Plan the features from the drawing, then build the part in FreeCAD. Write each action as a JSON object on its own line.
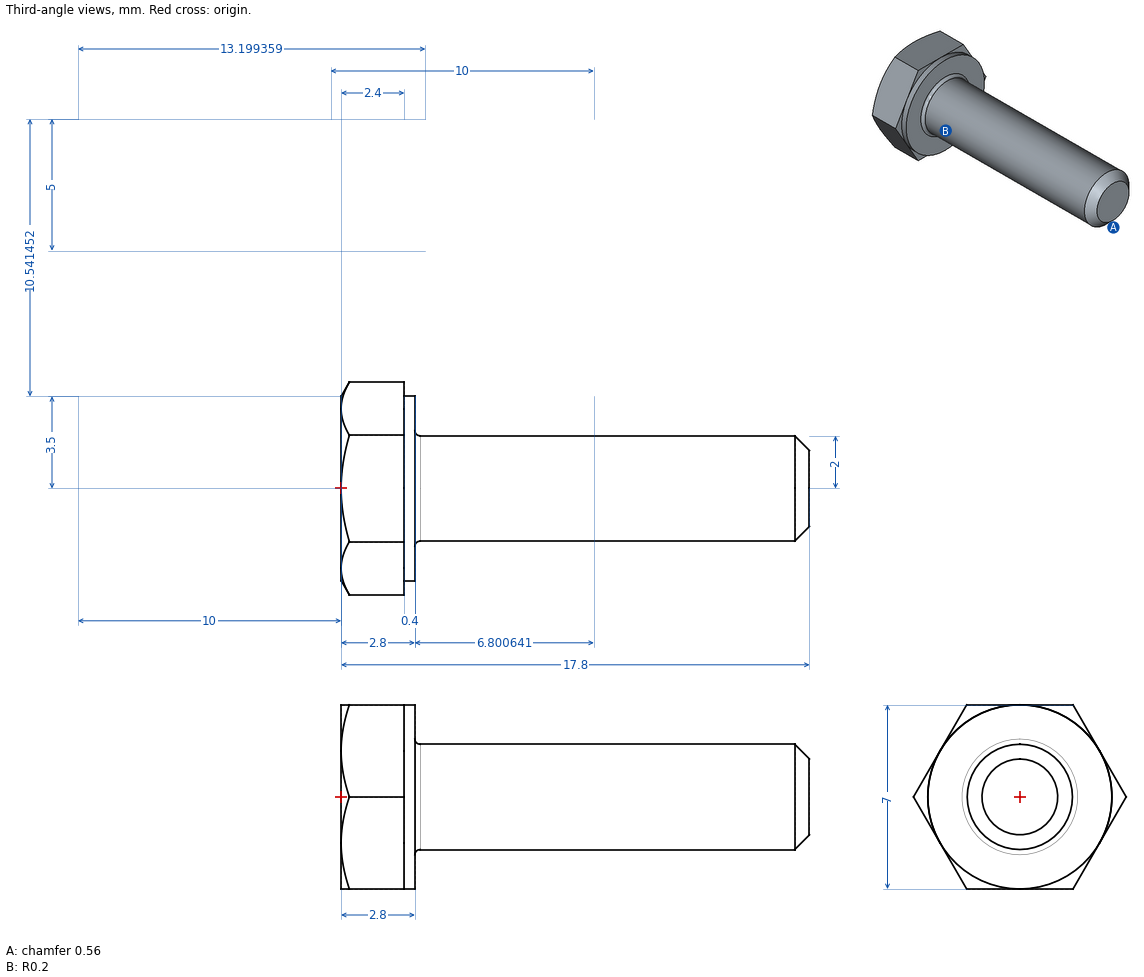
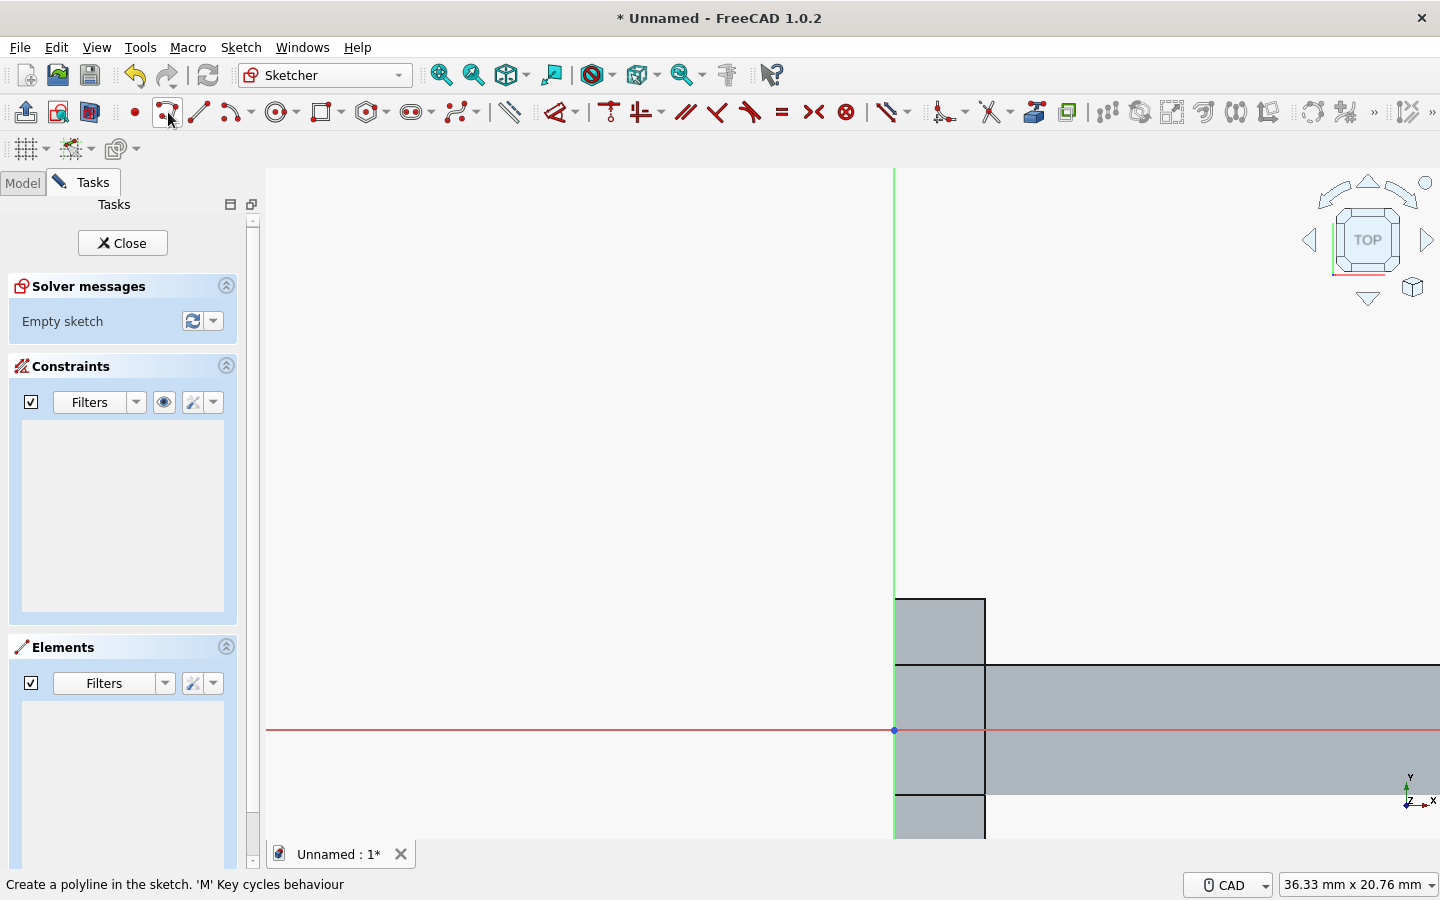
{"action": "left_click", "coordinate": [894, 617]}
{"action": "left_click", "coordinate": [998, 438]}
{"action": "left_click", "coordinate": [998, 276]}
{"action": "left_click", "coordinate": [571, 276]}
{"action": "left_click", "coordinate": [571, 617]}
{"action": "left_click", "coordinate": [894, 618]}
{"action": "key", "text": "Escape"}
{"action": "key", "text": "Escape"}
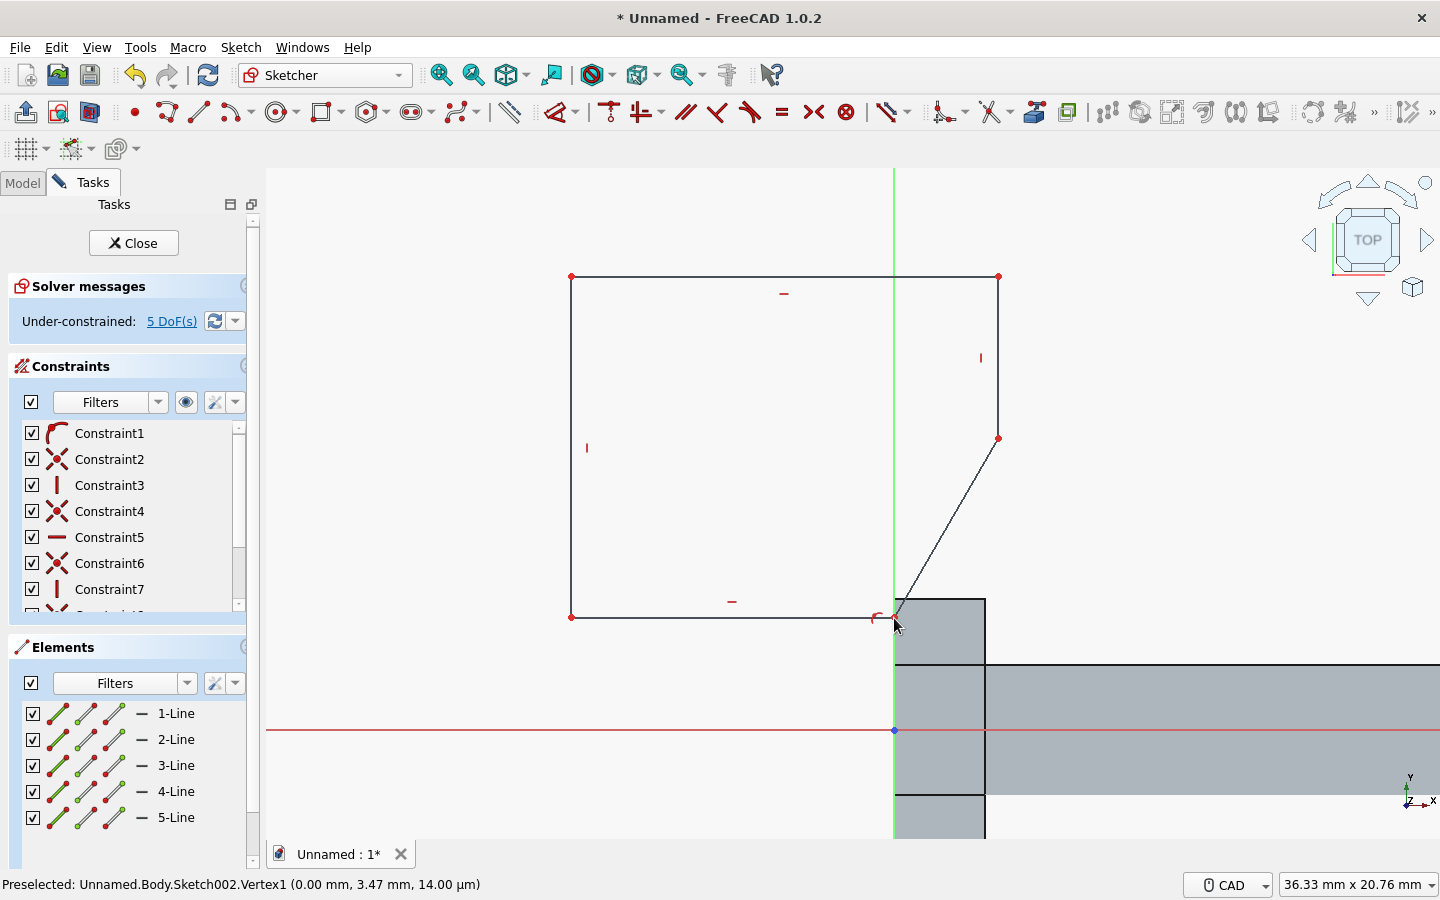
{"action": "key", "text": "d"}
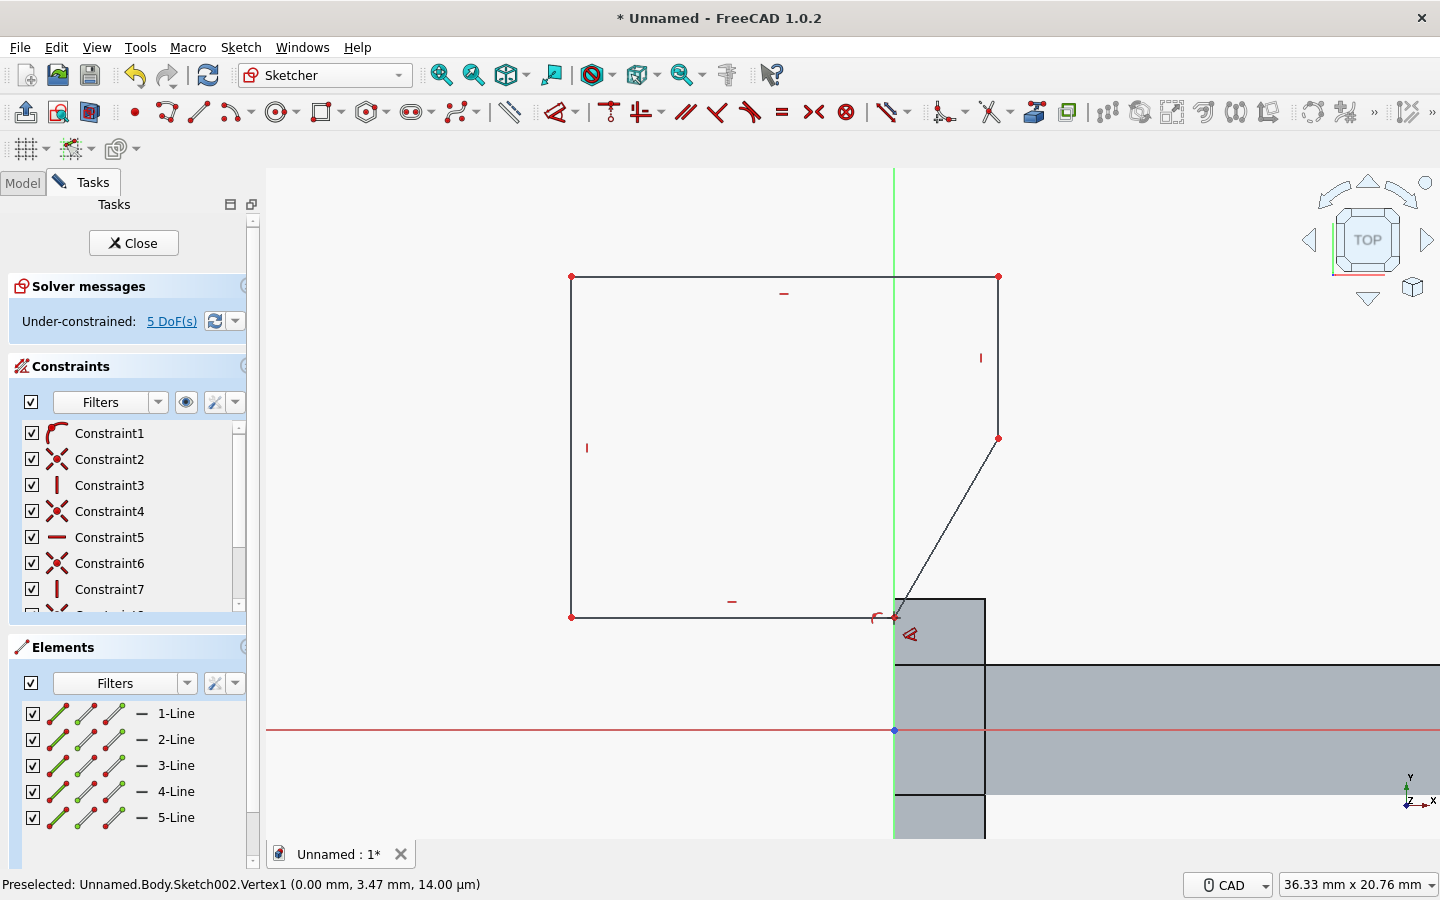
{"action": "left_click", "coordinate": [998, 390]}
{"action": "left_click", "coordinate": [1032, 358]}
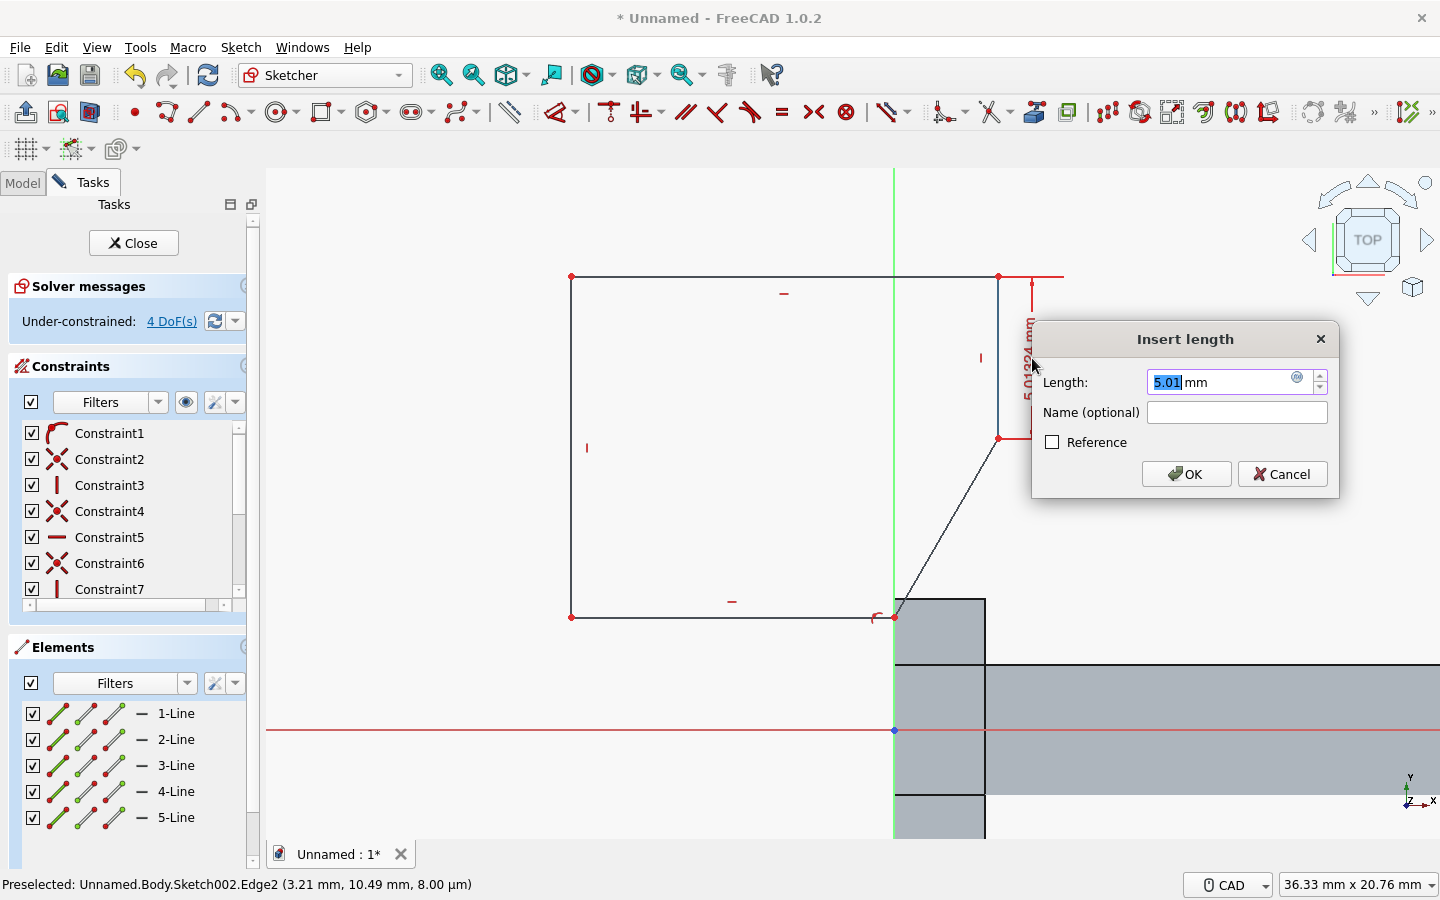
{"action": "type", "text": "5"}
{"action": "key", "text": "Return"}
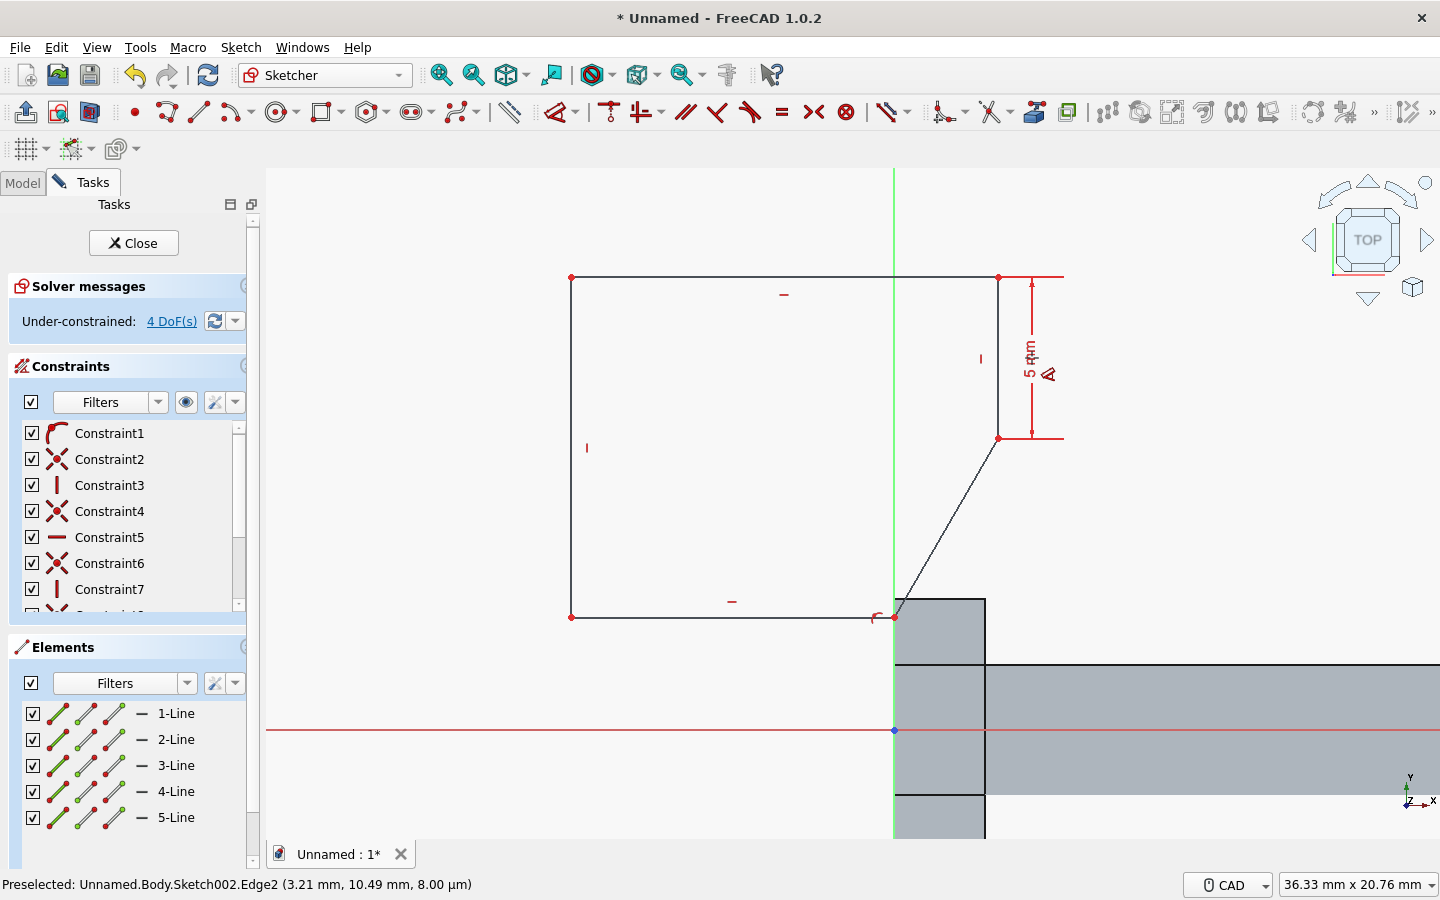
{"action": "left_click", "coordinate": [668, 618]}
{"action": "left_click", "coordinate": [733, 652]}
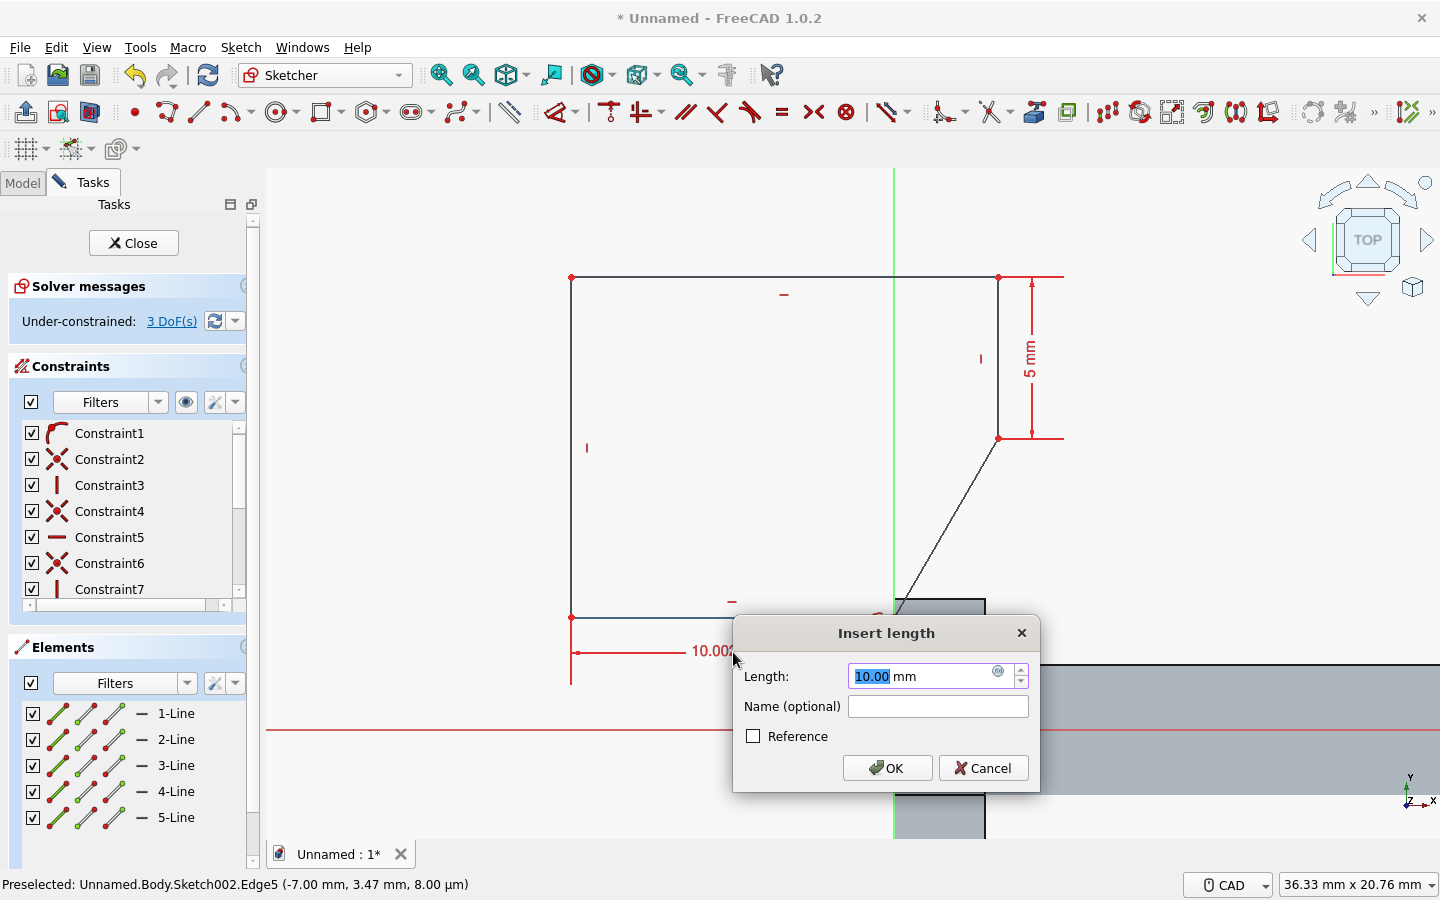
{"action": "type", "text": "10"}
{"action": "key", "text": "Return"}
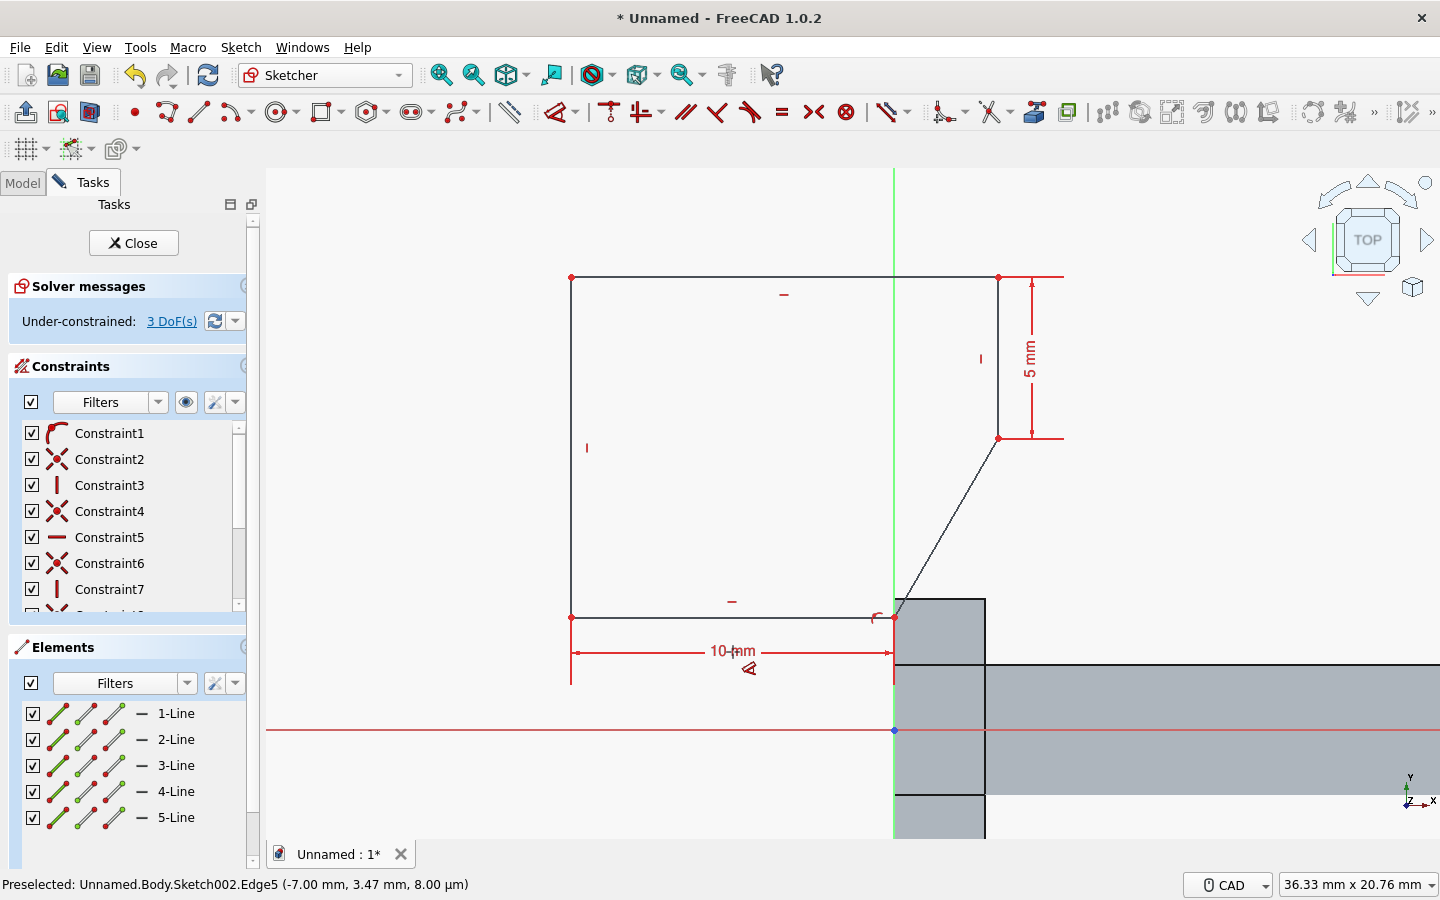
{"action": "left_click", "coordinate": [894, 618]}
{"action": "left_click", "coordinate": [928, 674]}